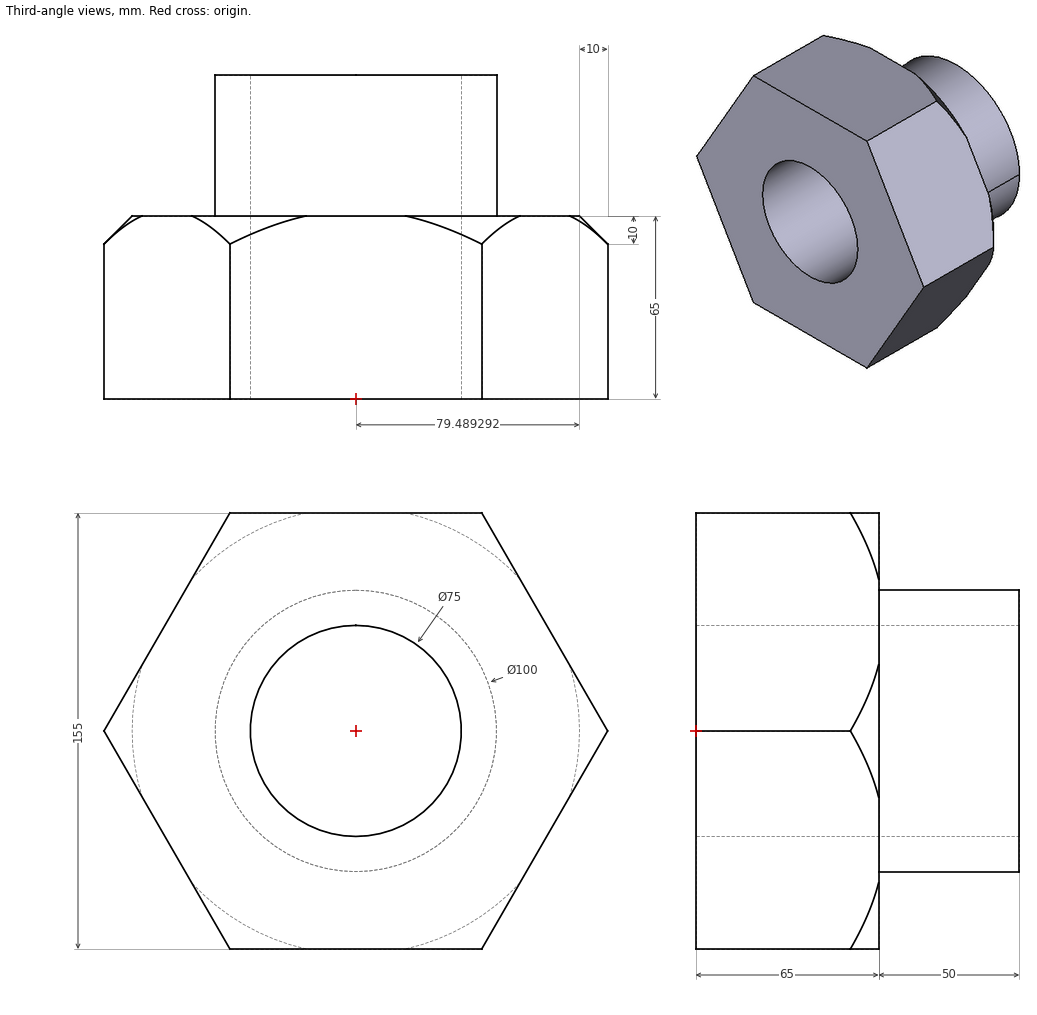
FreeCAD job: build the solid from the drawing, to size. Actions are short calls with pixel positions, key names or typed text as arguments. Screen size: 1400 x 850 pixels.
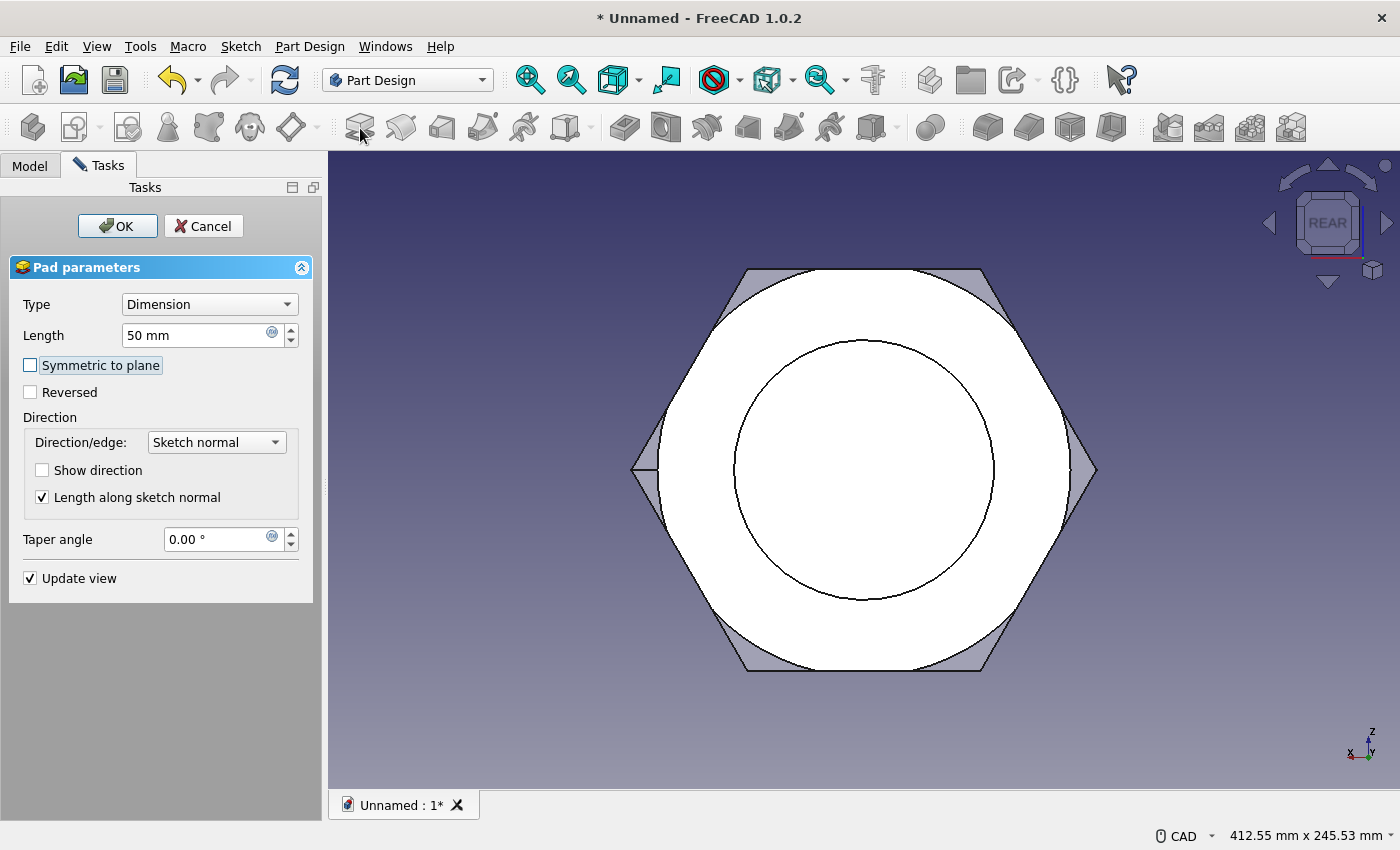
click(118, 226)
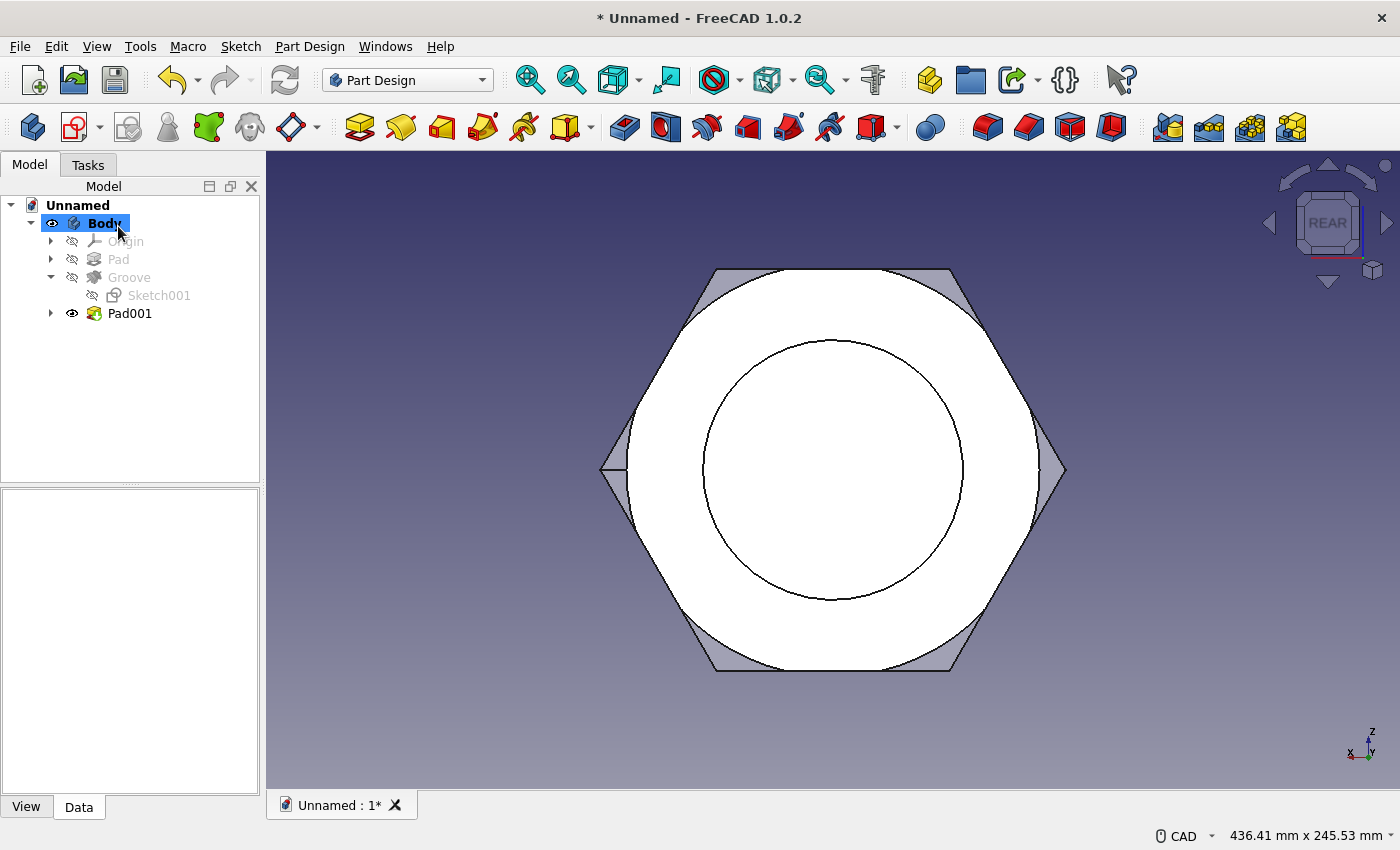
click(833, 469)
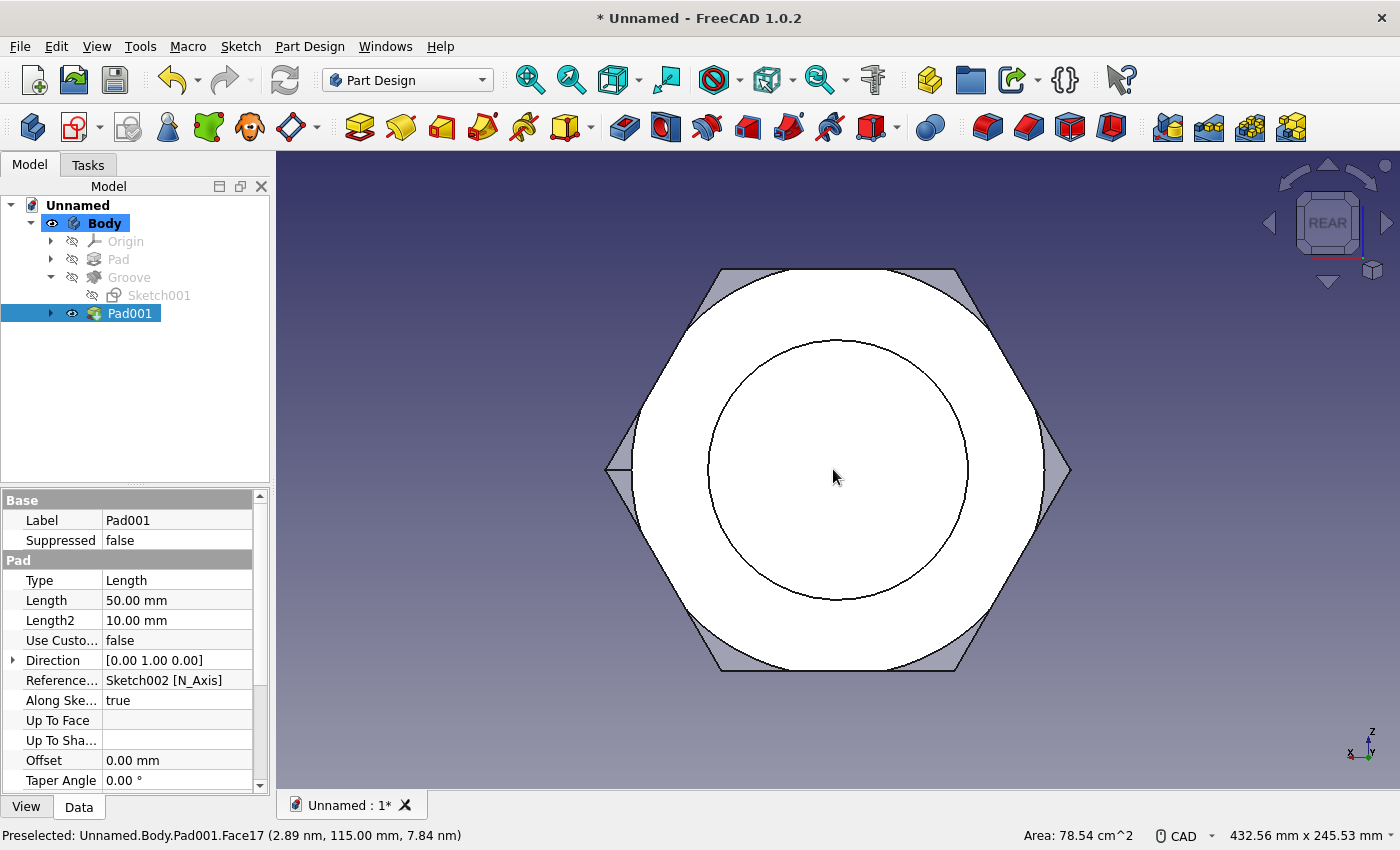
click(74, 128)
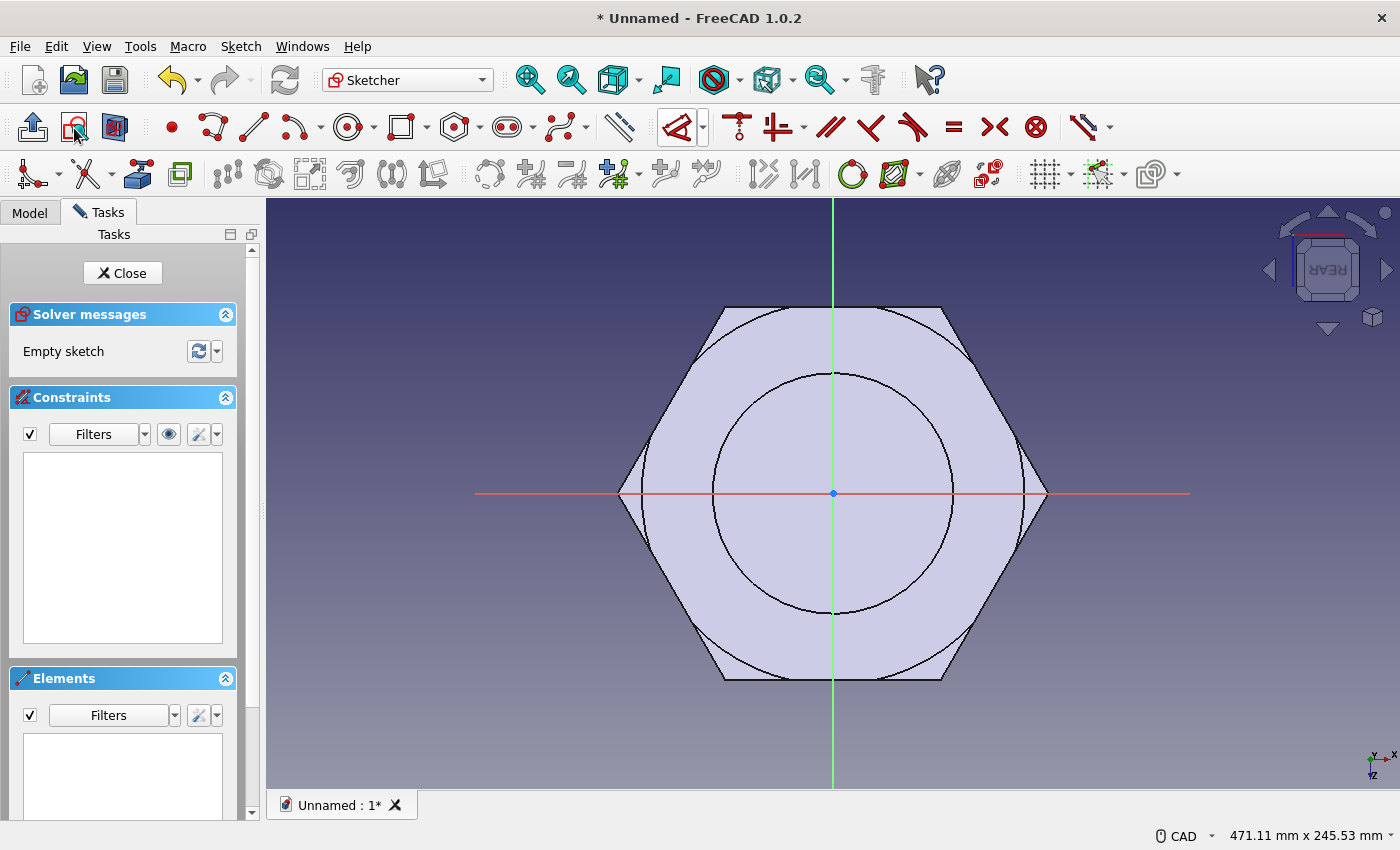
scroll(889, 493, up, 4)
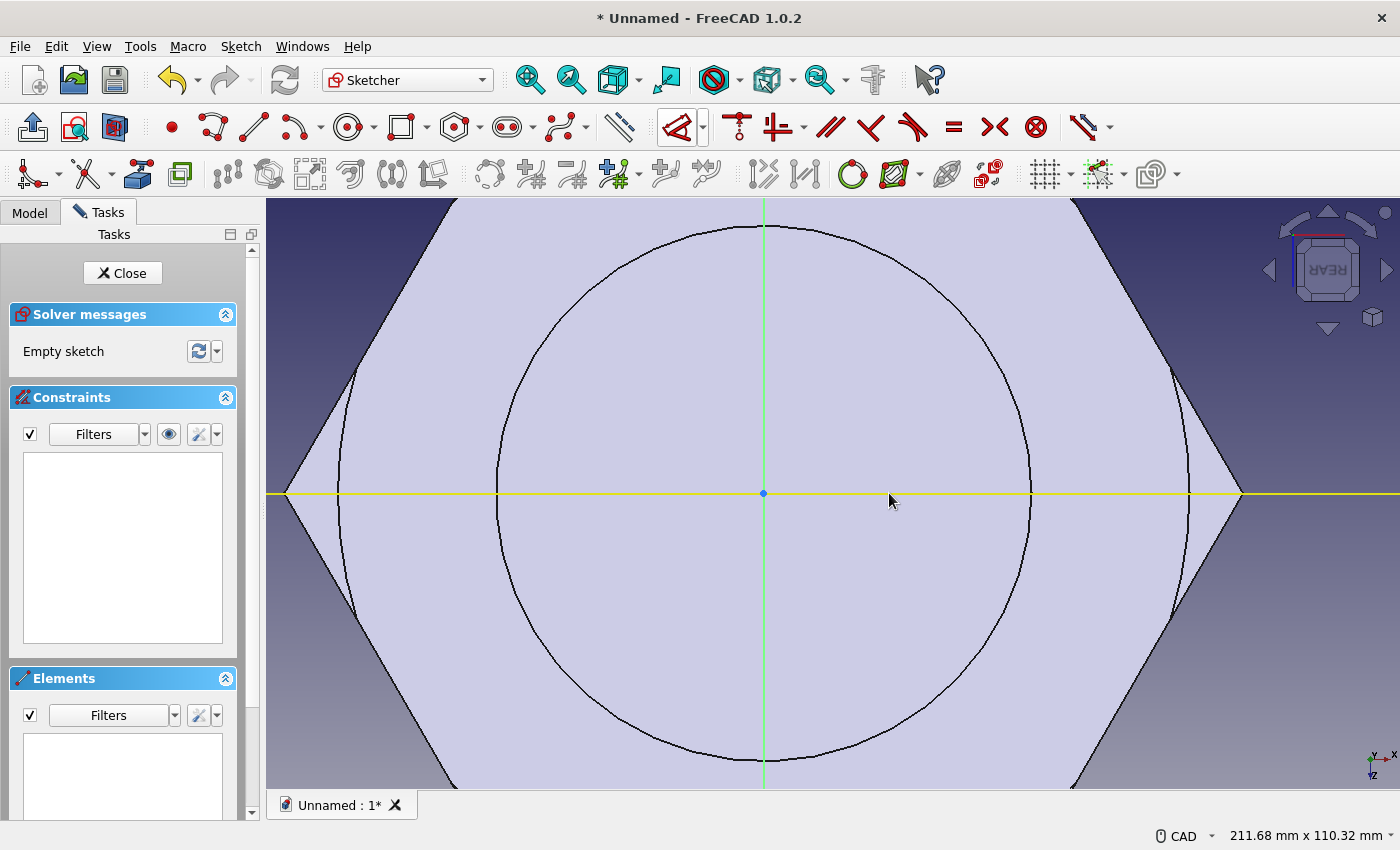
click(348, 128)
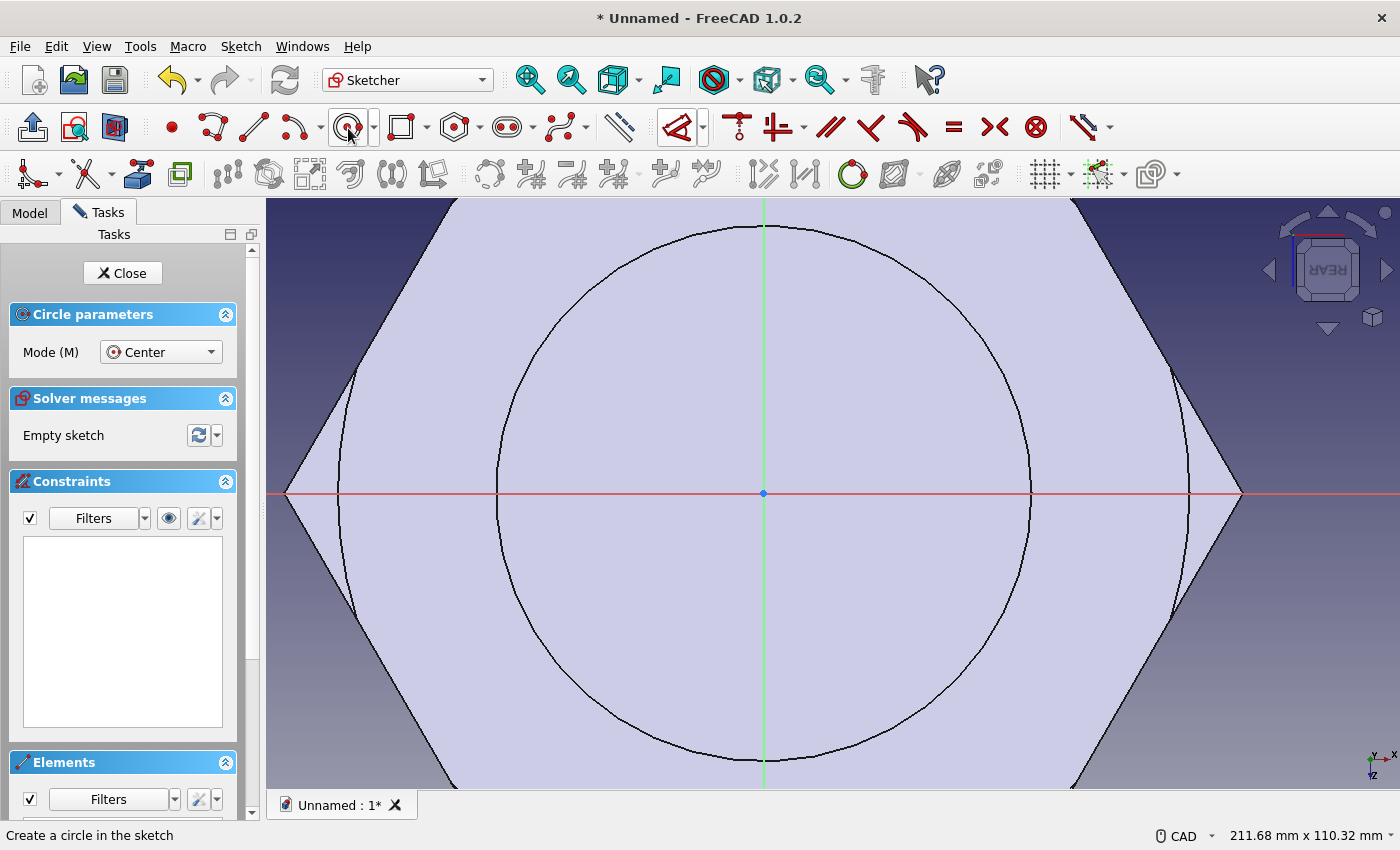
click(764, 493)
click(906, 351)
key(Escape)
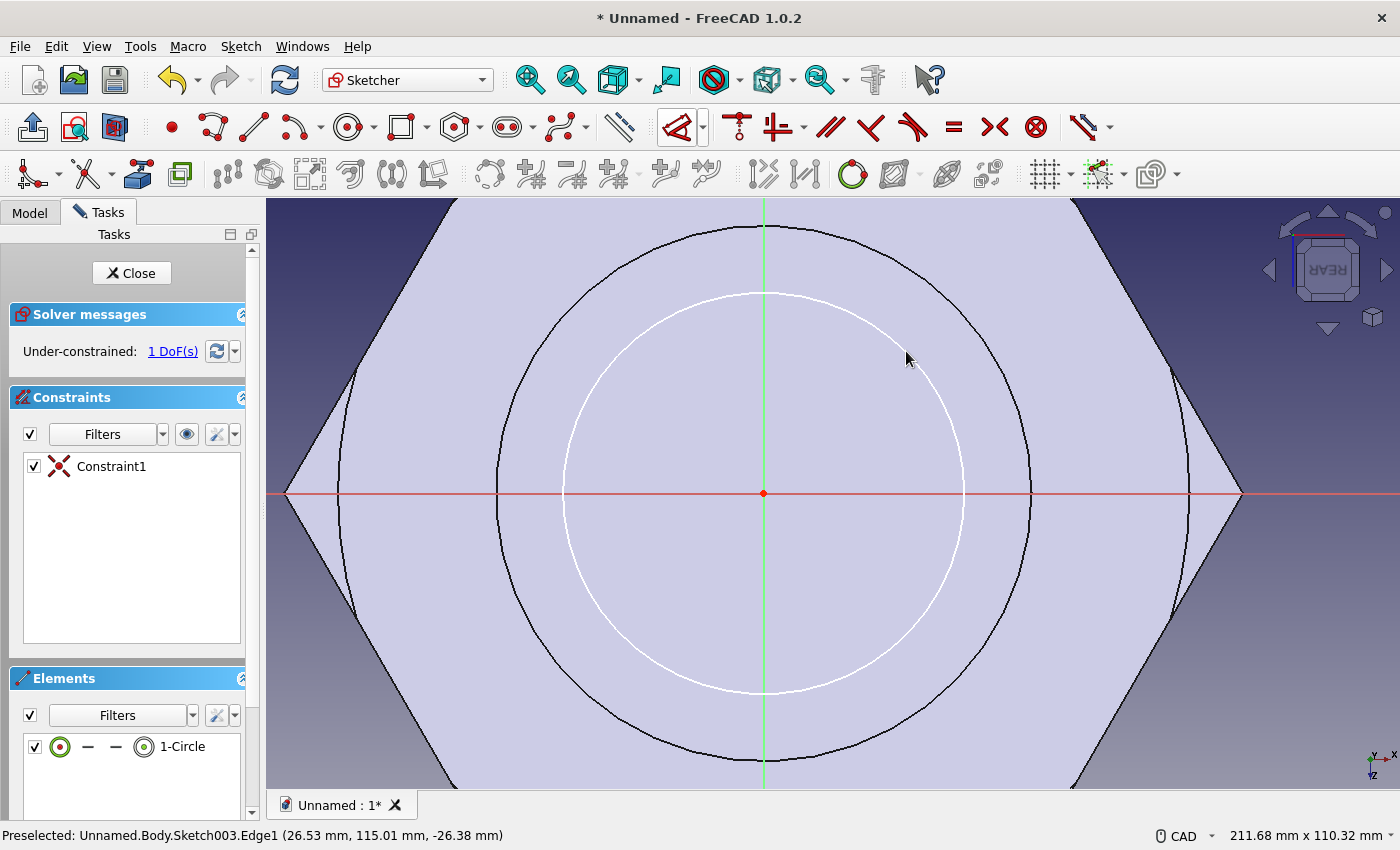
click(905, 351)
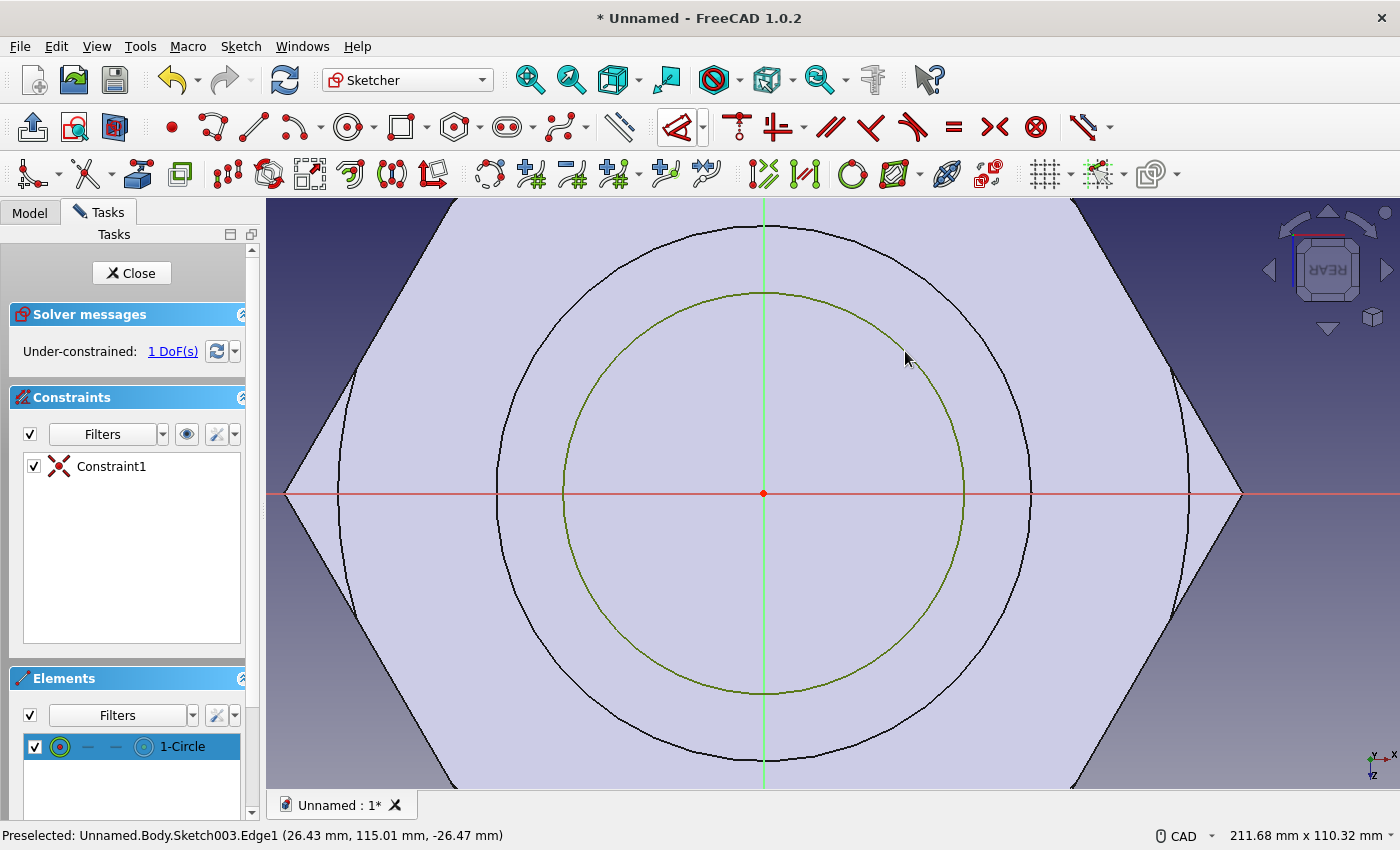
click(702, 128)